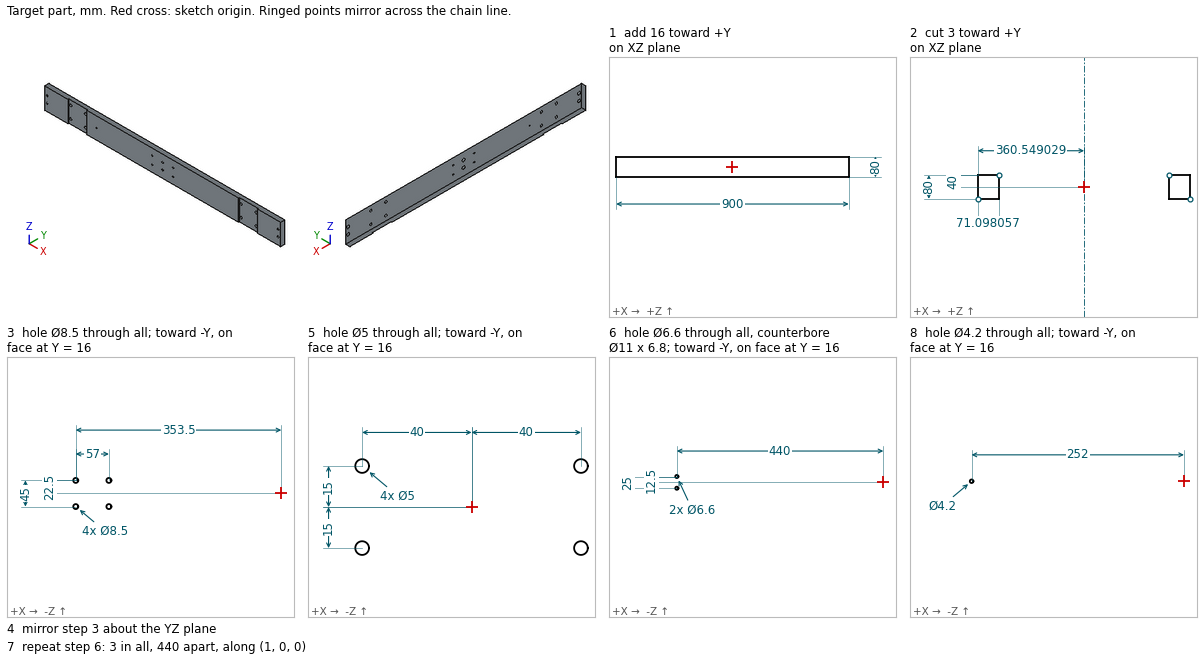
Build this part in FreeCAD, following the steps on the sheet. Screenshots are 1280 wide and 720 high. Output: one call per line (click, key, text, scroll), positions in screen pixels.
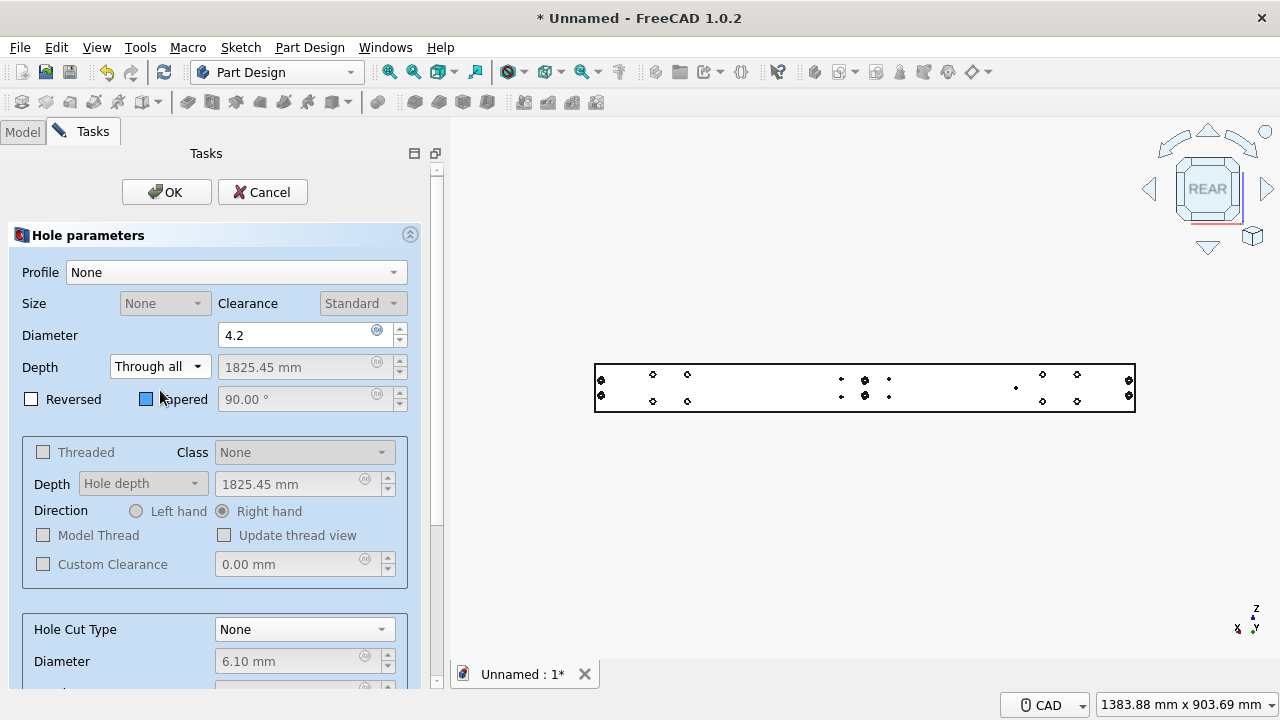
click(167, 192)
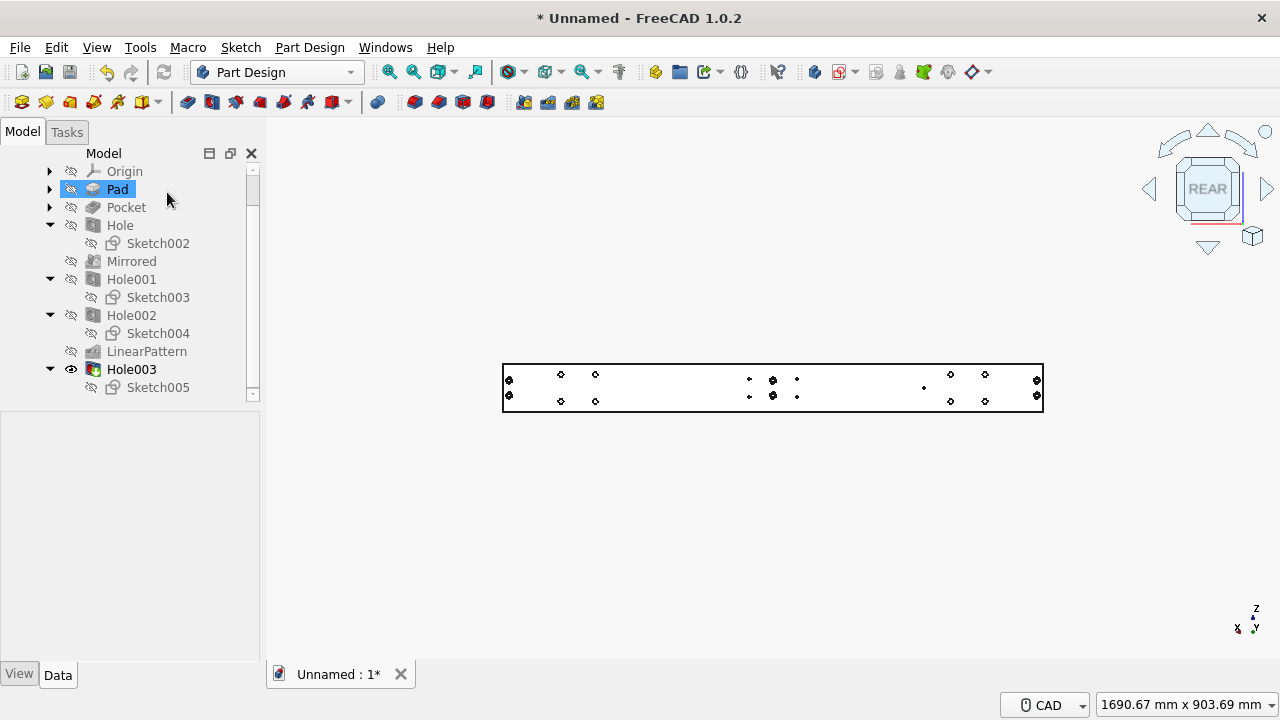
key(0)